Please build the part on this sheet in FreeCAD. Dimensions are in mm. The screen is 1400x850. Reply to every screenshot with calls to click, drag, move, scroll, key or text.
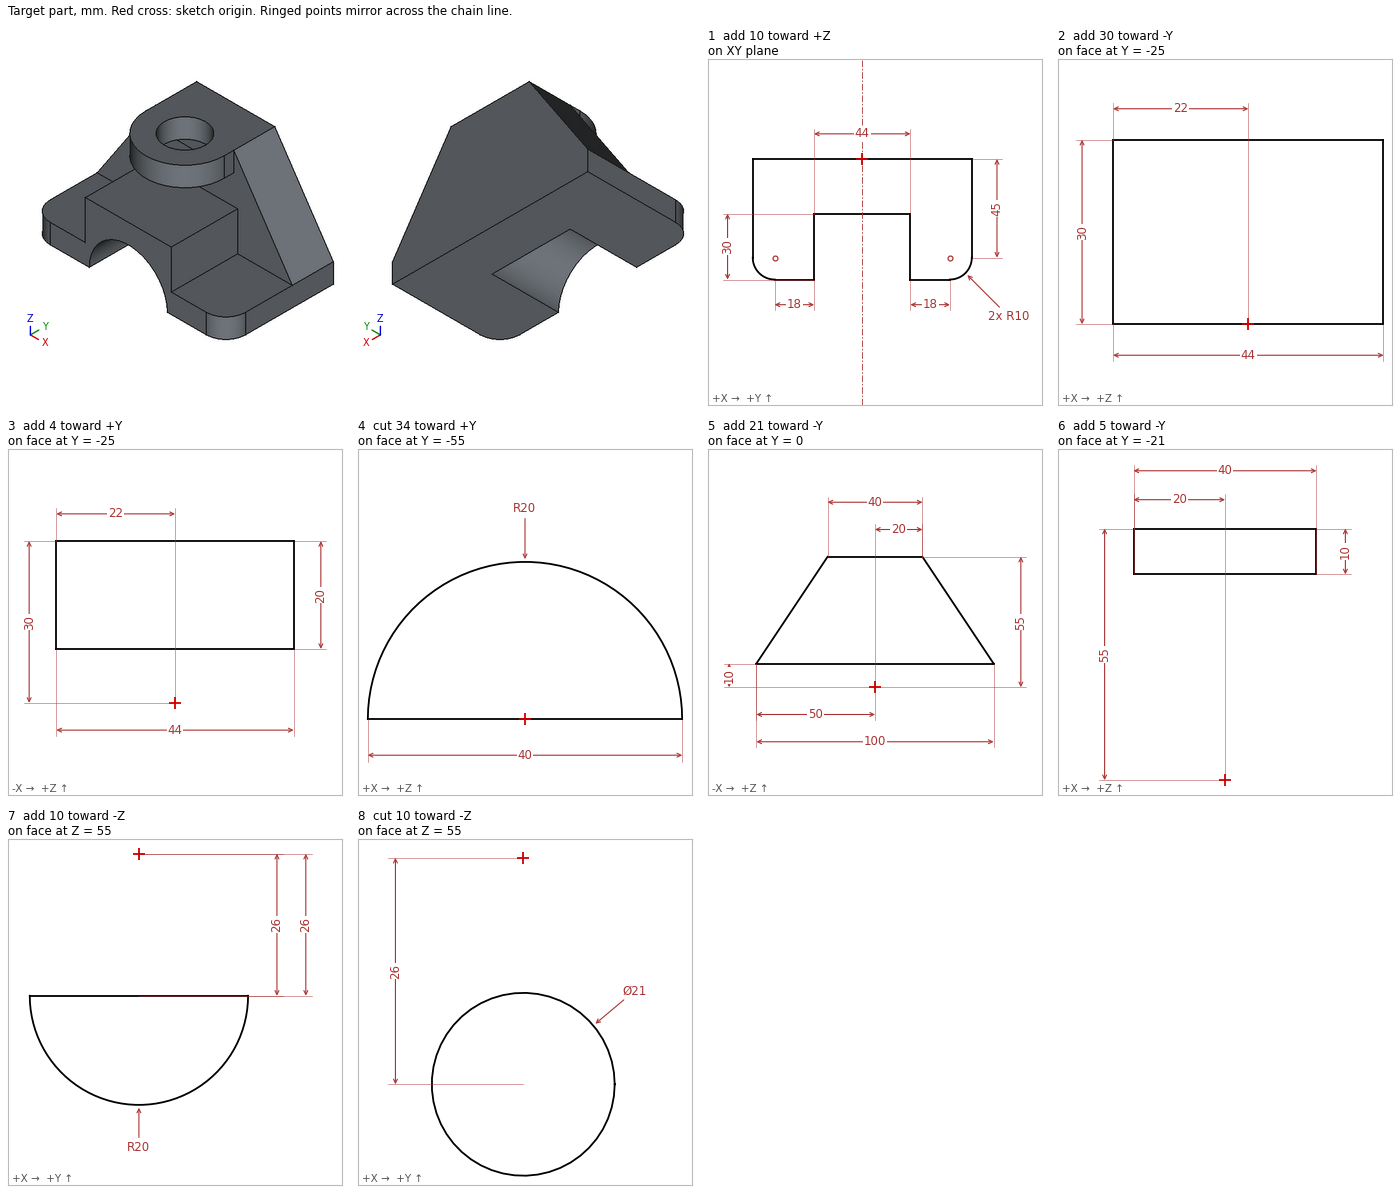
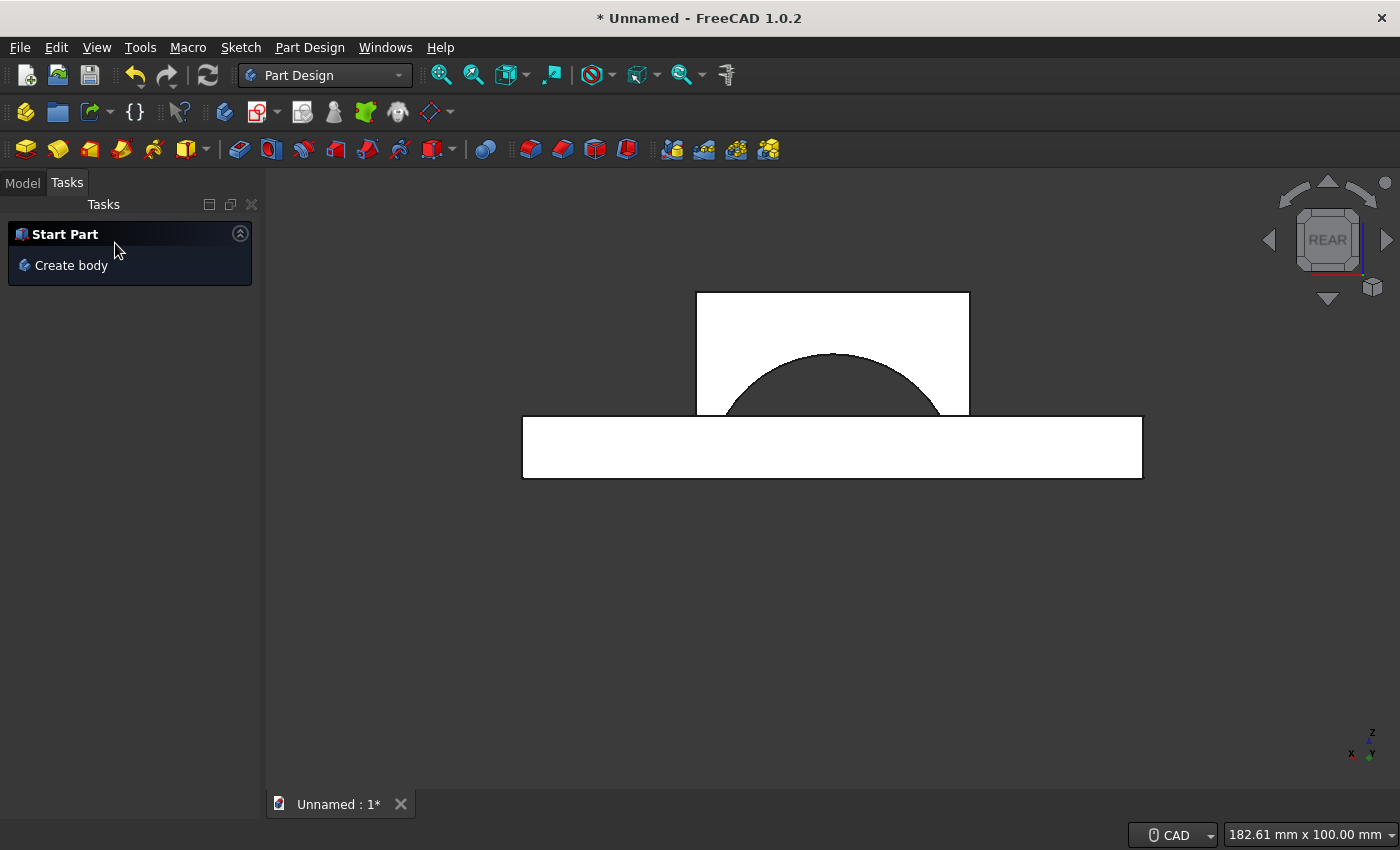
click(567, 446)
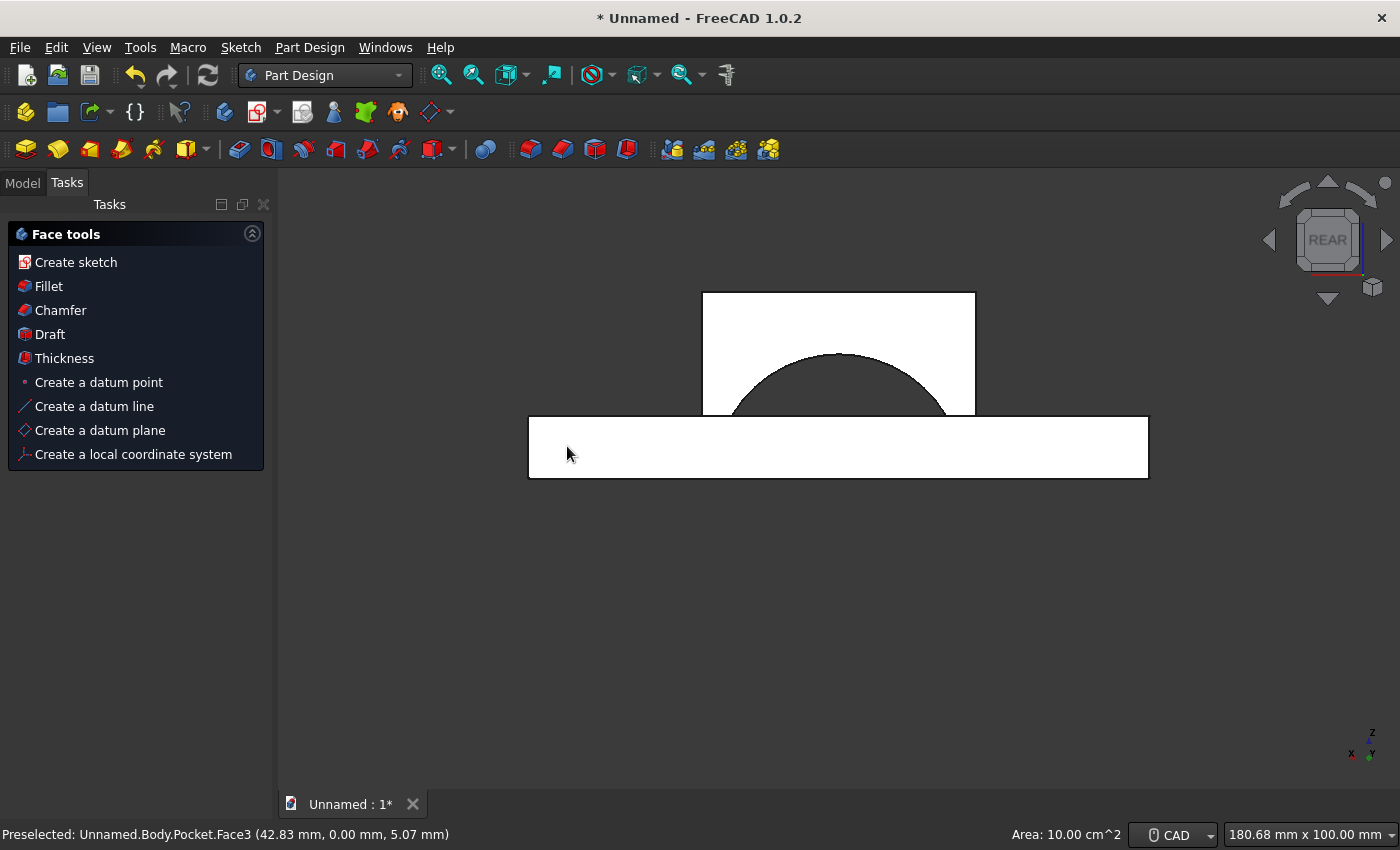
click(258, 112)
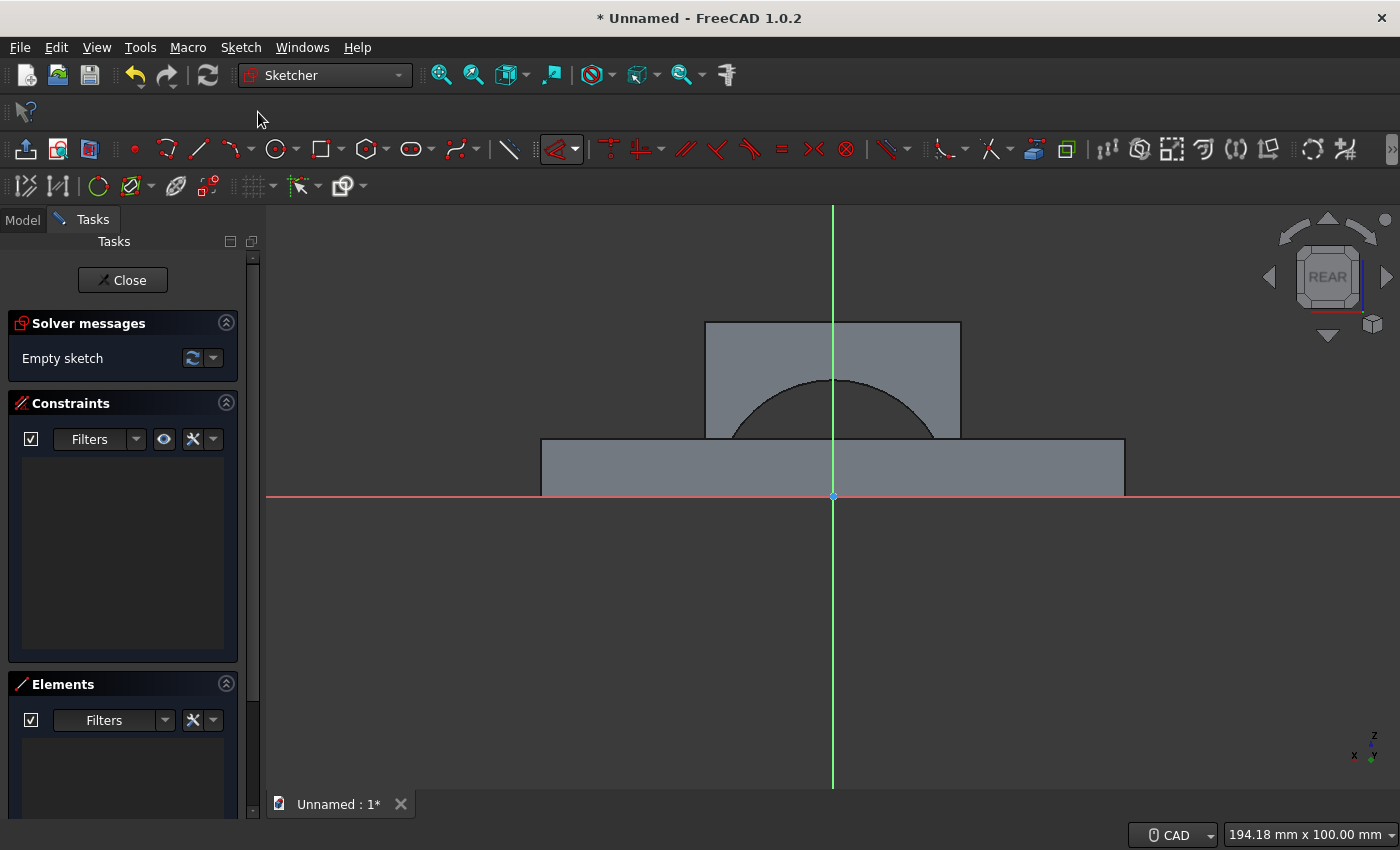
scroll(455, 761, down, 1)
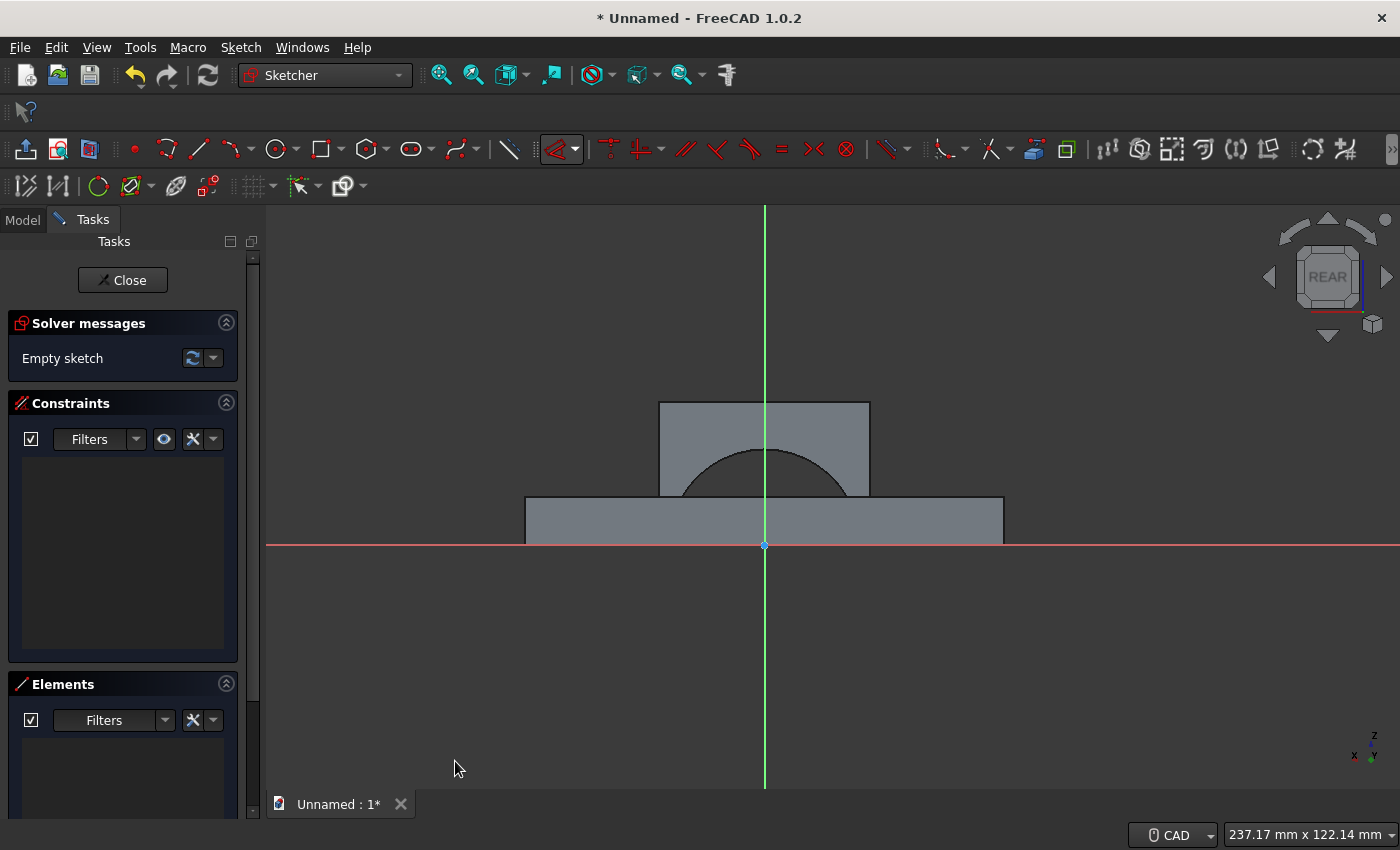
scroll(765, 244, up, 2)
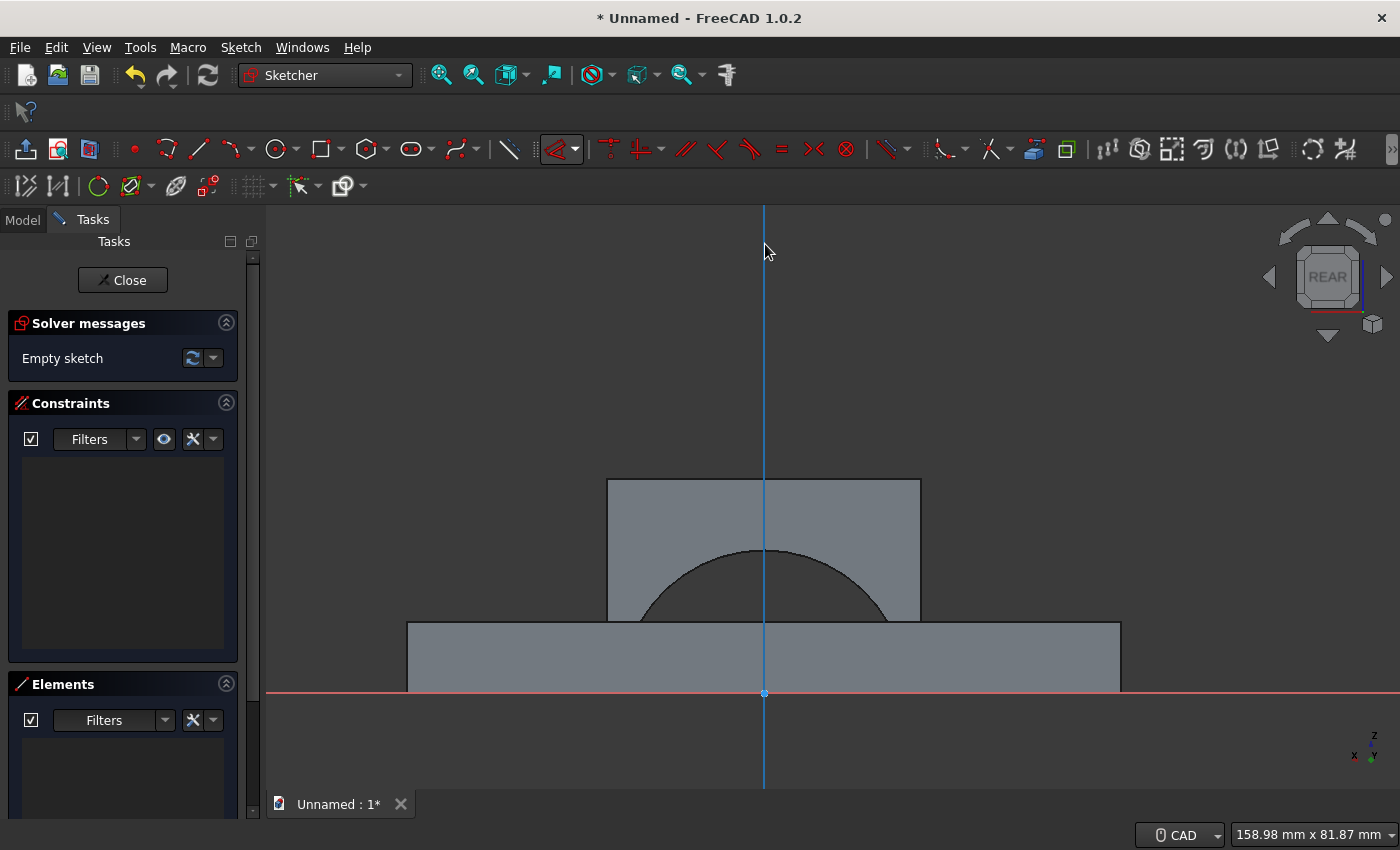
click(168, 150)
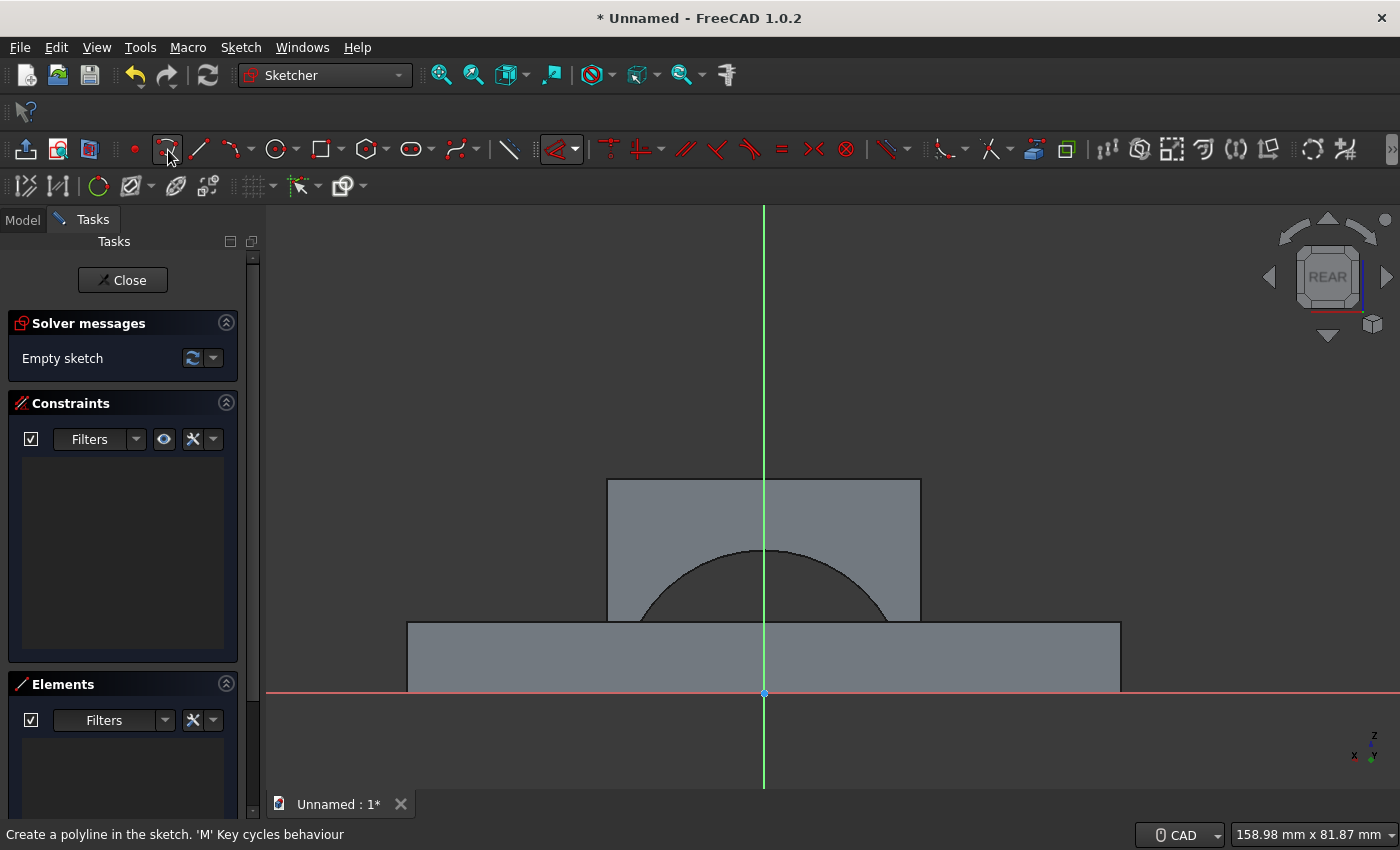
click(407, 622)
click(1121, 622)
click(907, 301)
click(621, 301)
click(407, 623)
key(Escape)
key(Escape)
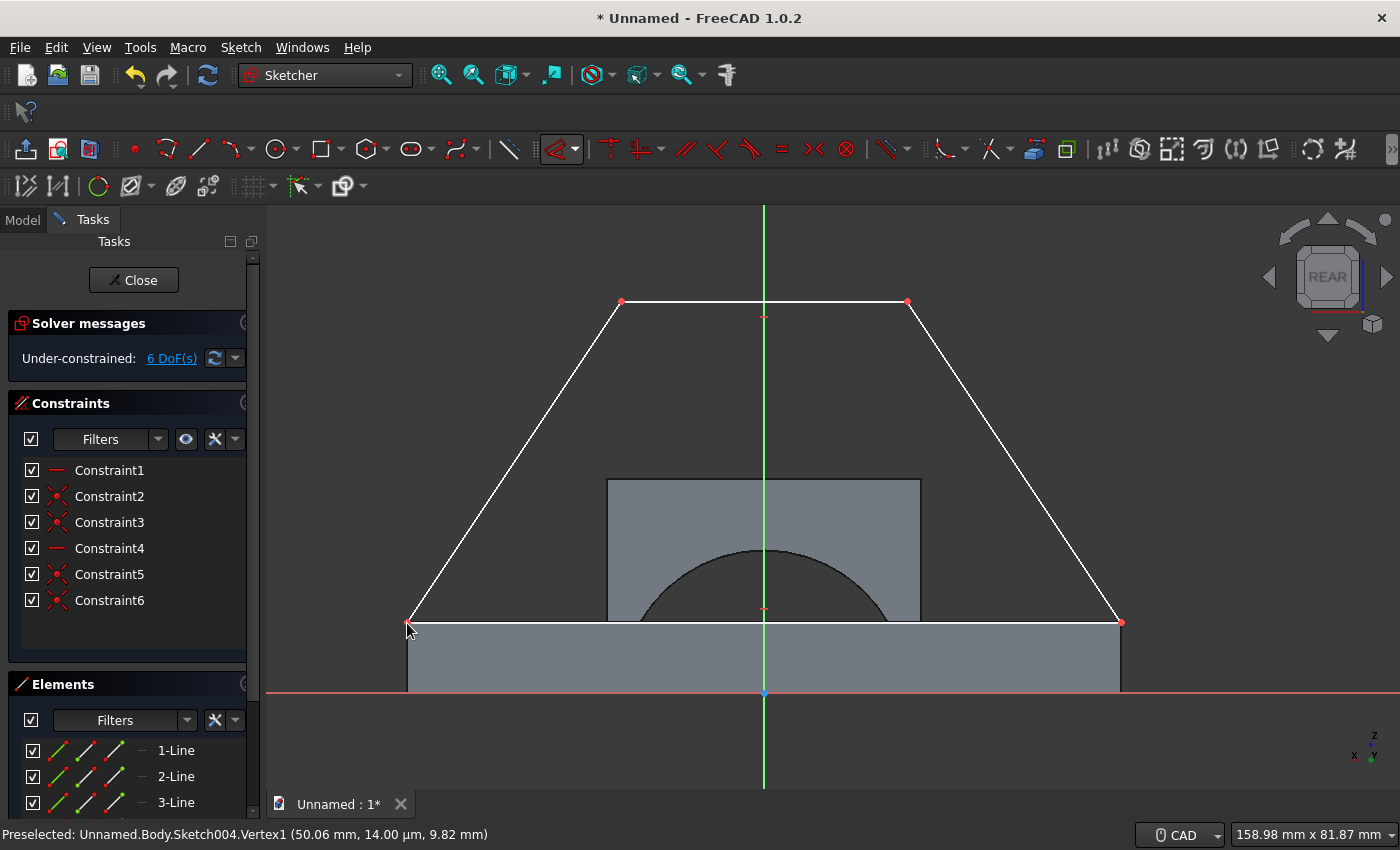
click(821, 302)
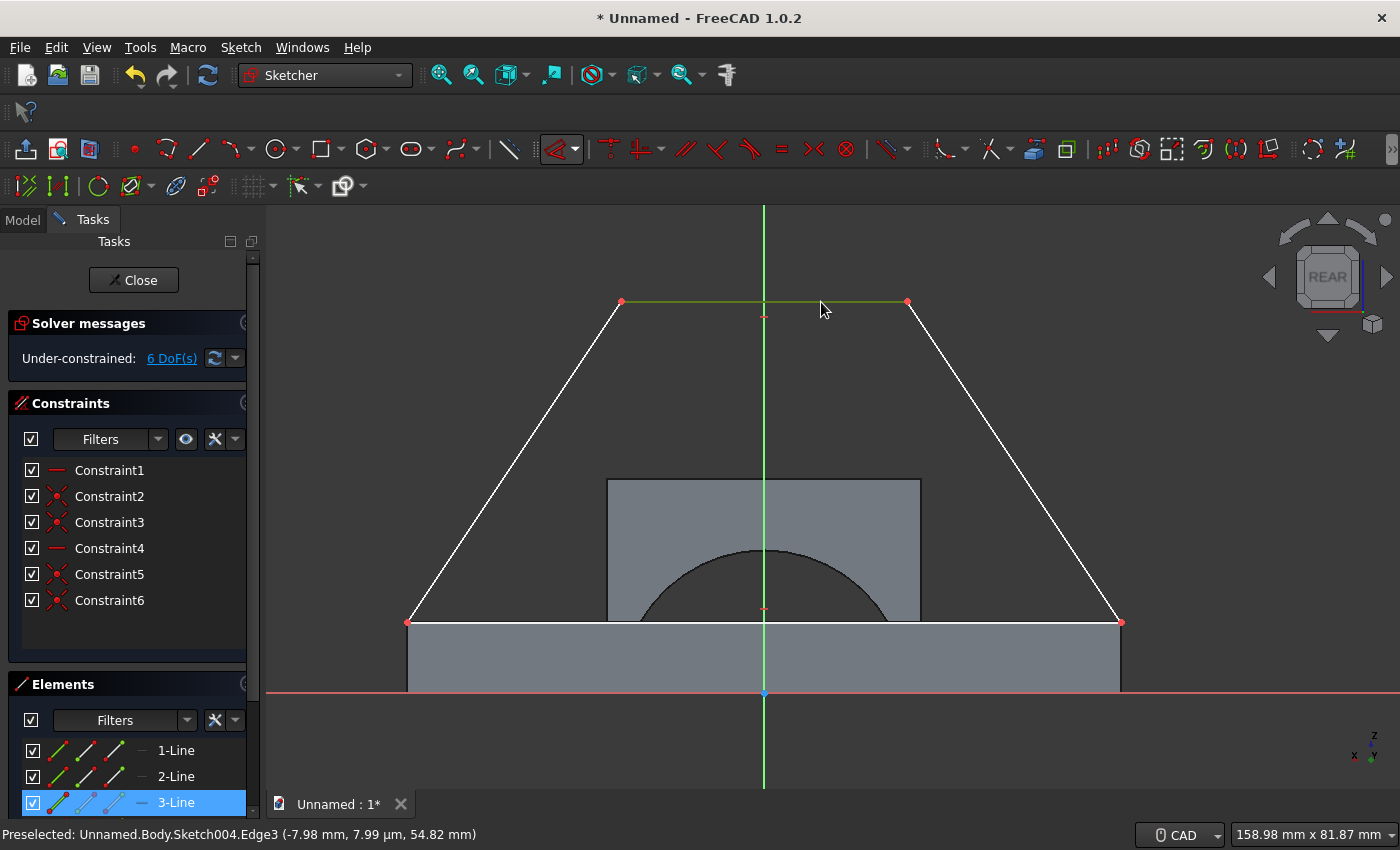
key(l)